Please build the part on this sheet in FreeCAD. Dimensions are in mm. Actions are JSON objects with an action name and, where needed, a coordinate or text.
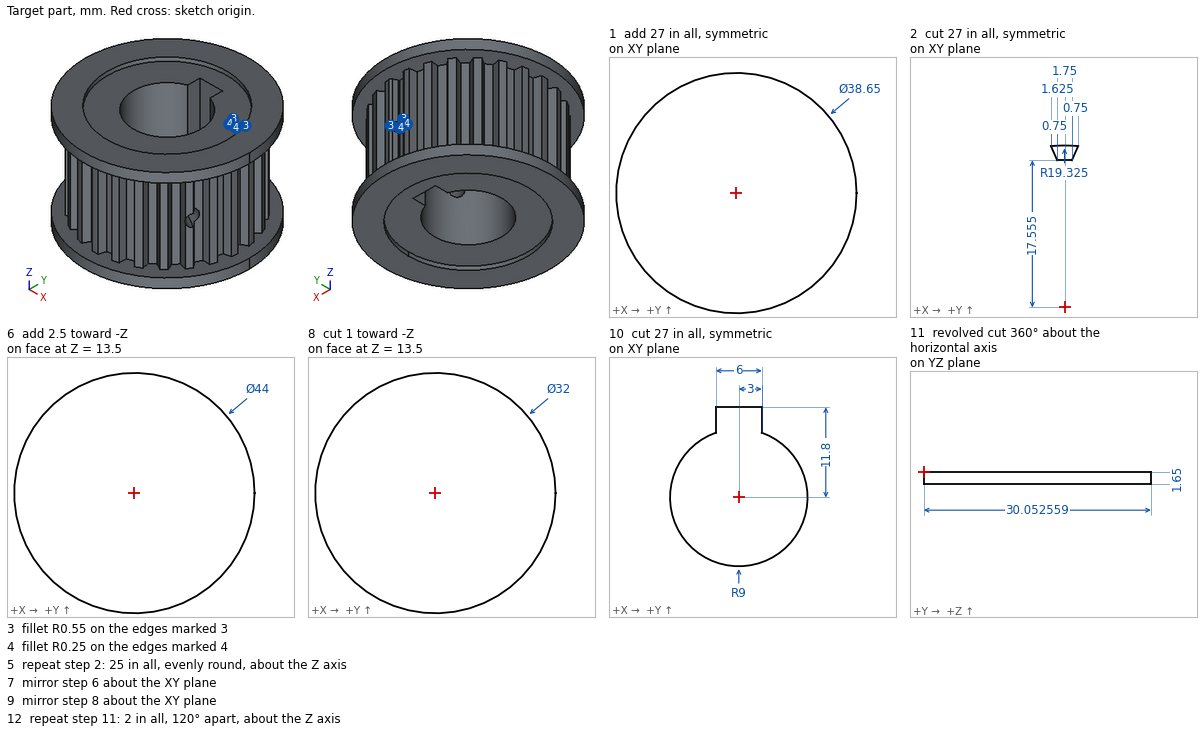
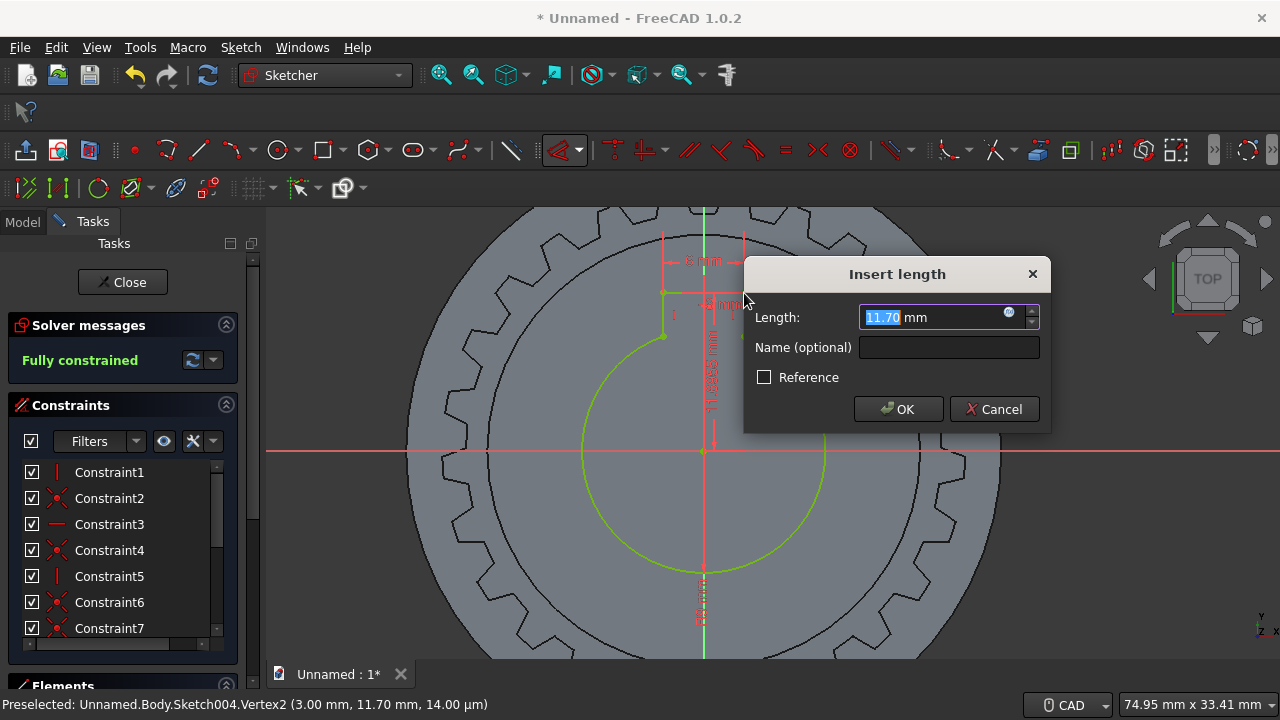
{"action": "type", "text": "11.8"}
{"action": "key", "text": "Return"}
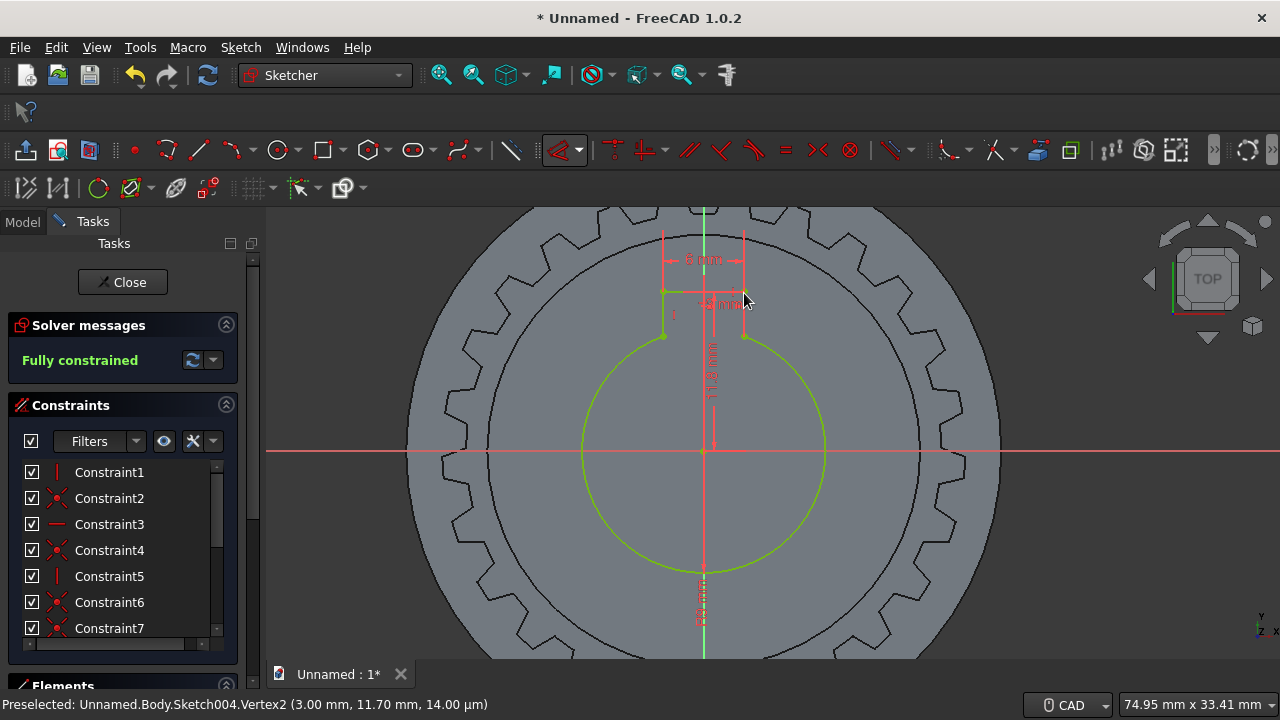
{"action": "left_click", "coordinate": [123, 282]}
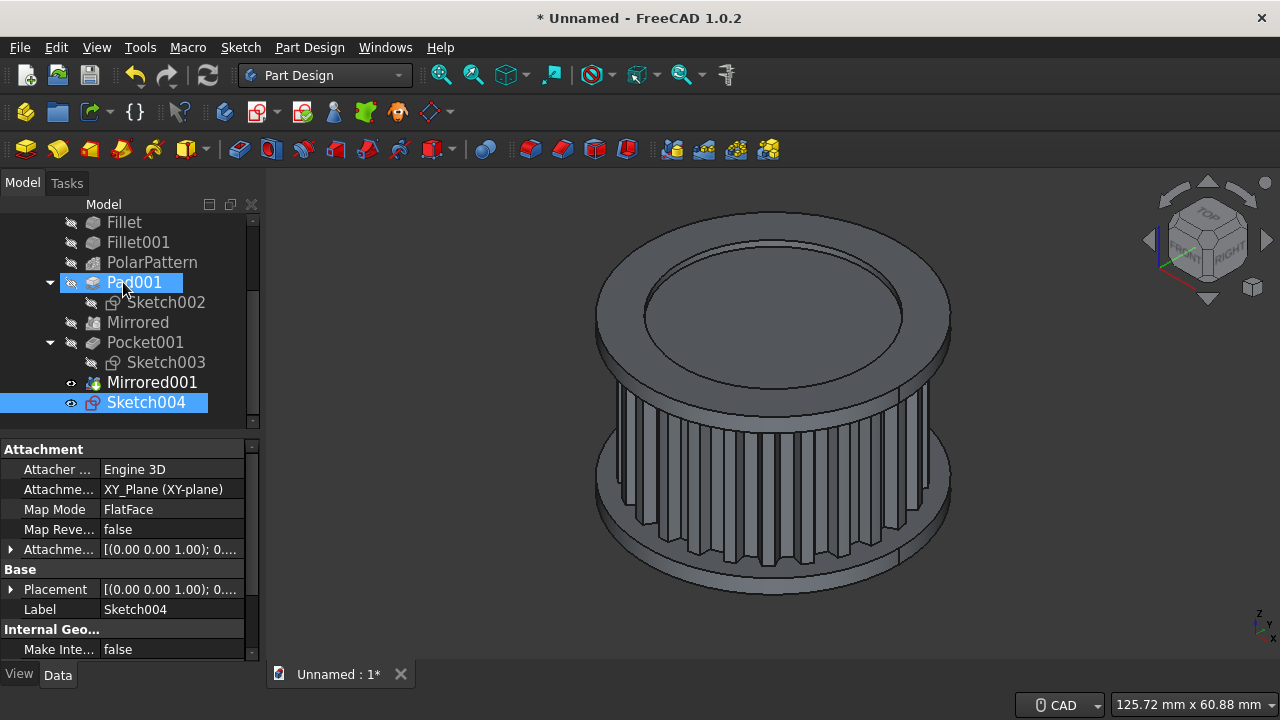
{"action": "left_click", "coordinate": [240, 150]}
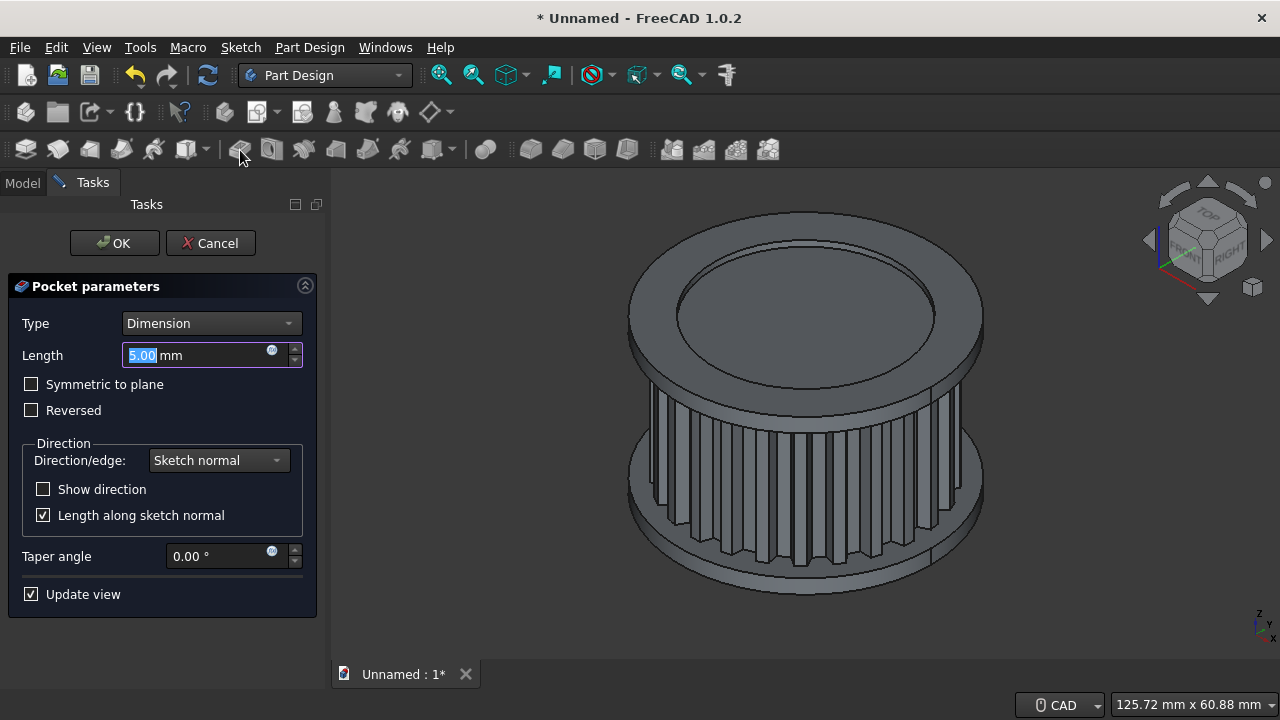
{"action": "type", "text": "27"}
{"action": "key", "text": "Tab"}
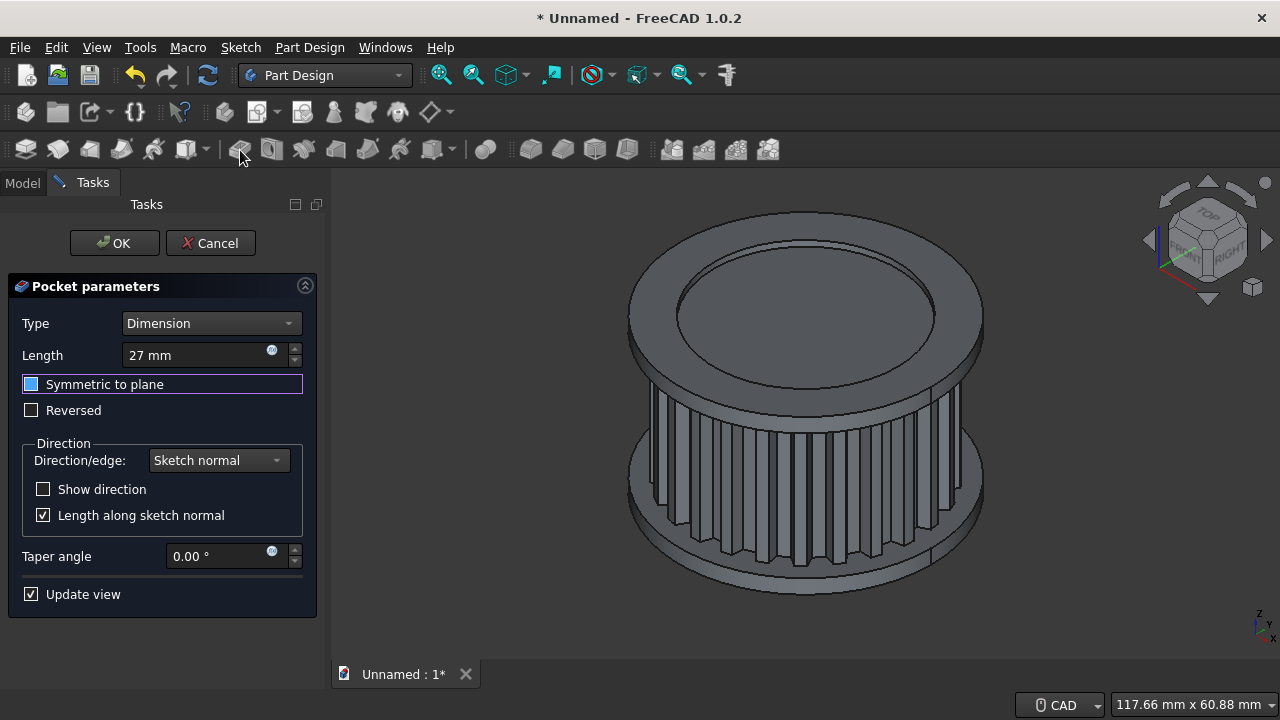
{"action": "left_click", "coordinate": [30, 384]}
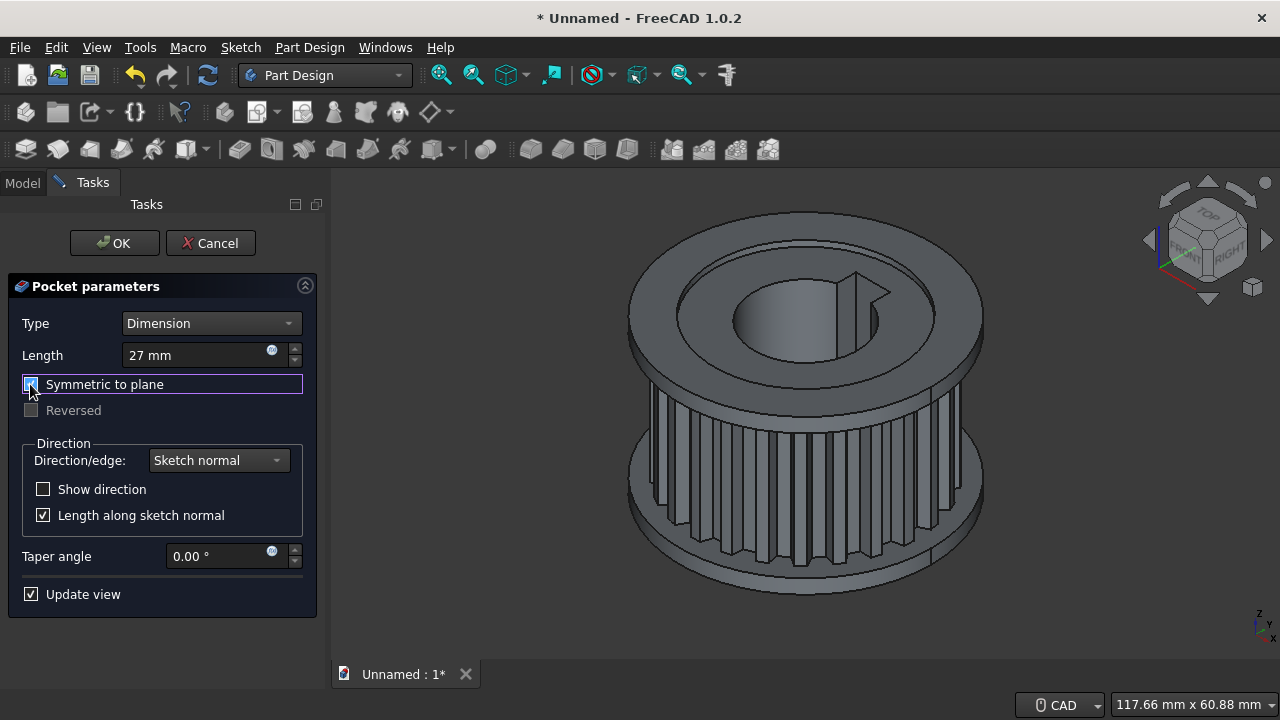
{"action": "left_click", "coordinate": [115, 243]}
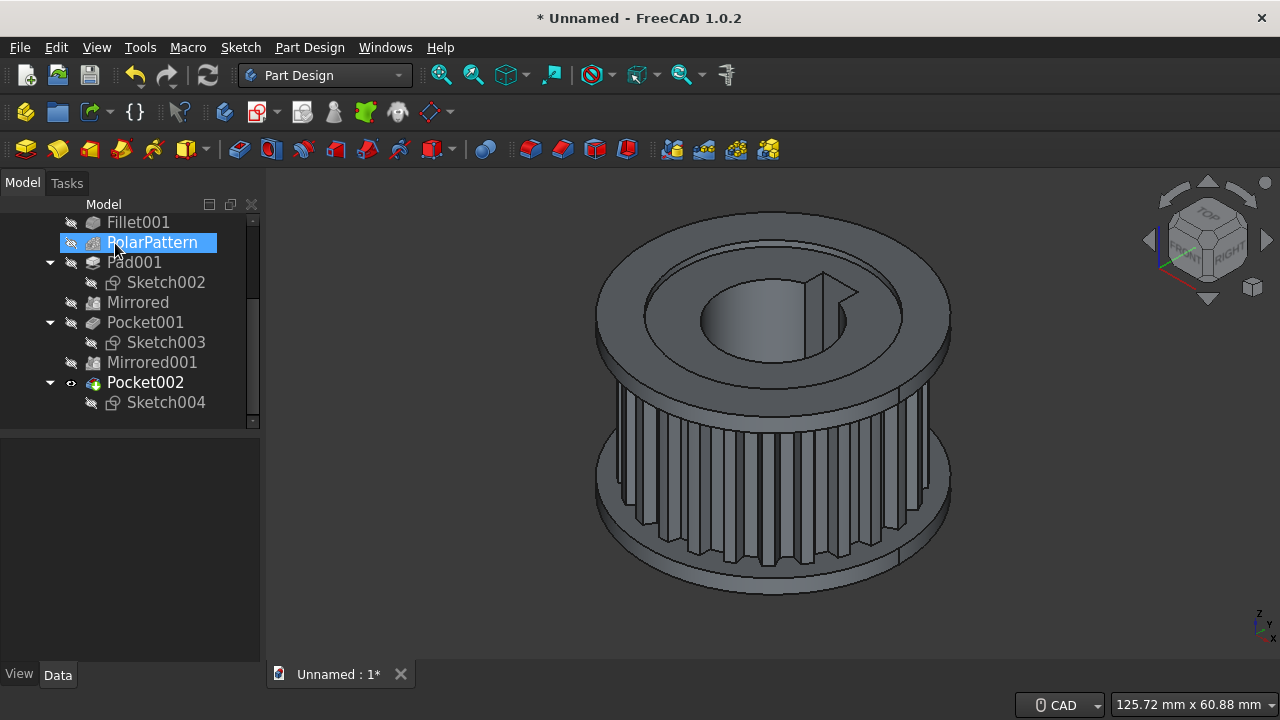
{"action": "left_click", "coordinate": [258, 112]}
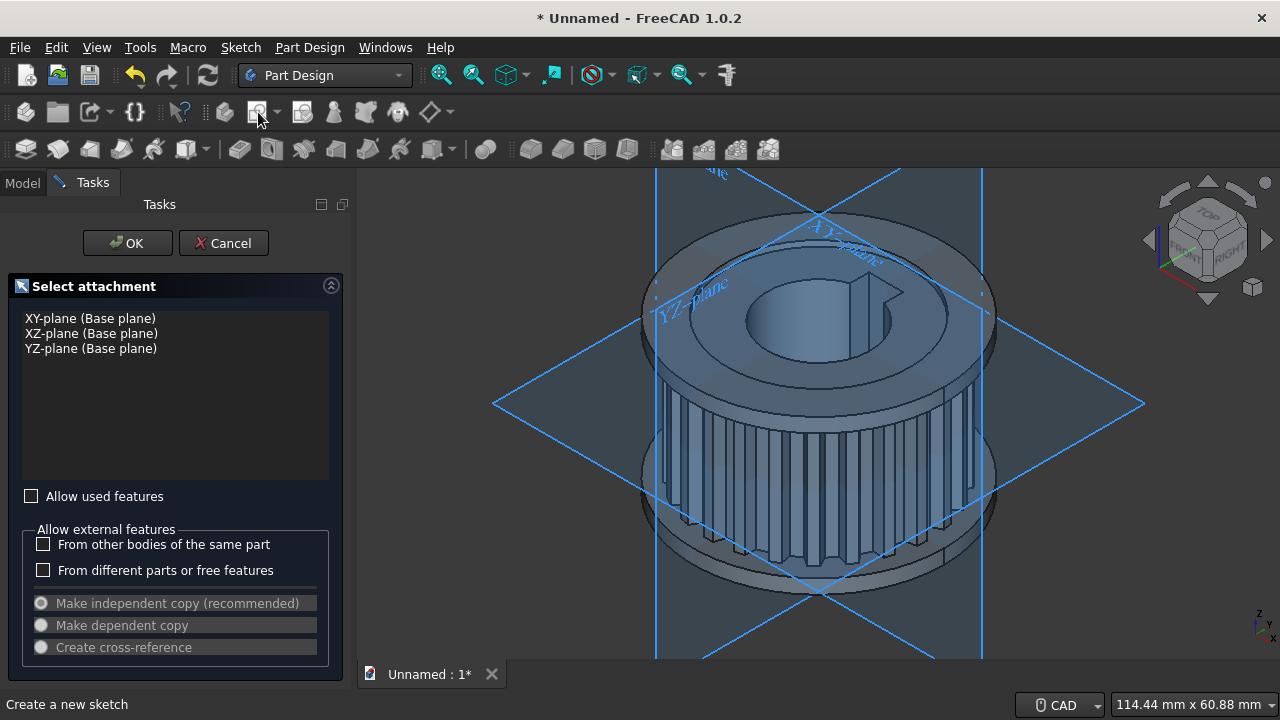
{"action": "left_click", "coordinate": [82, 348]}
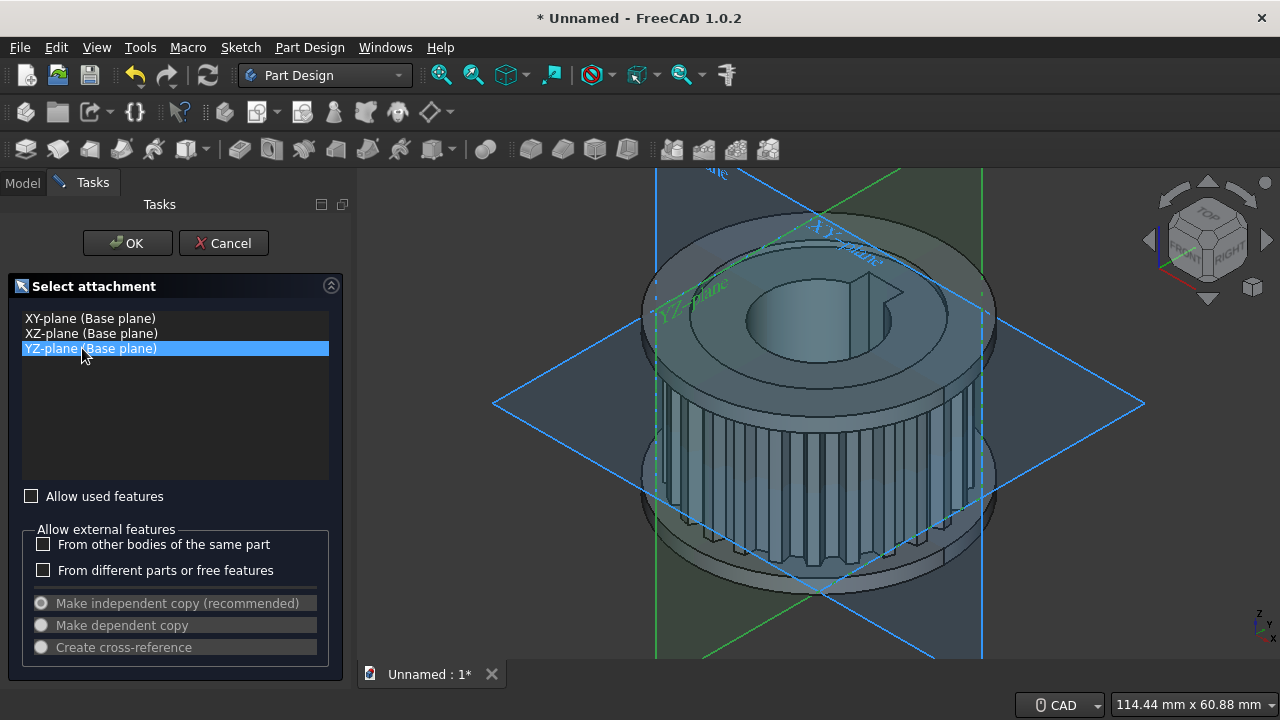
{"action": "left_click", "coordinate": [128, 243]}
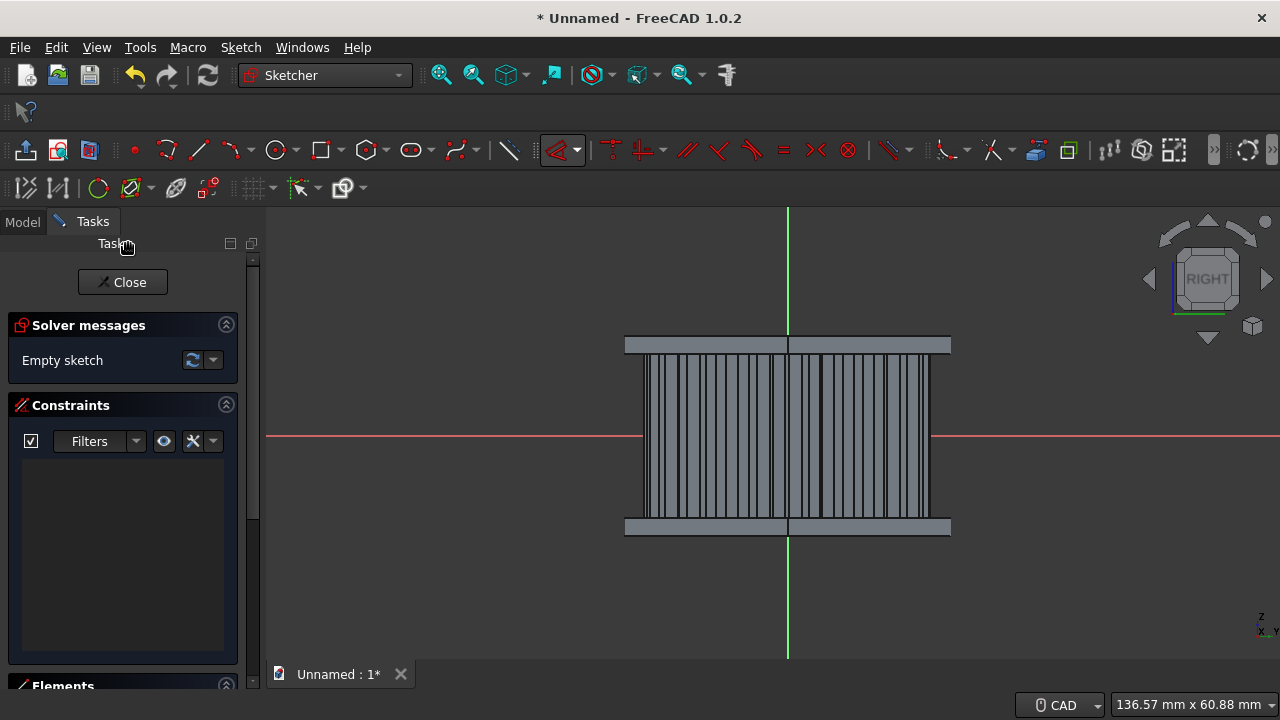
{"action": "left_click", "coordinate": [90, 150]}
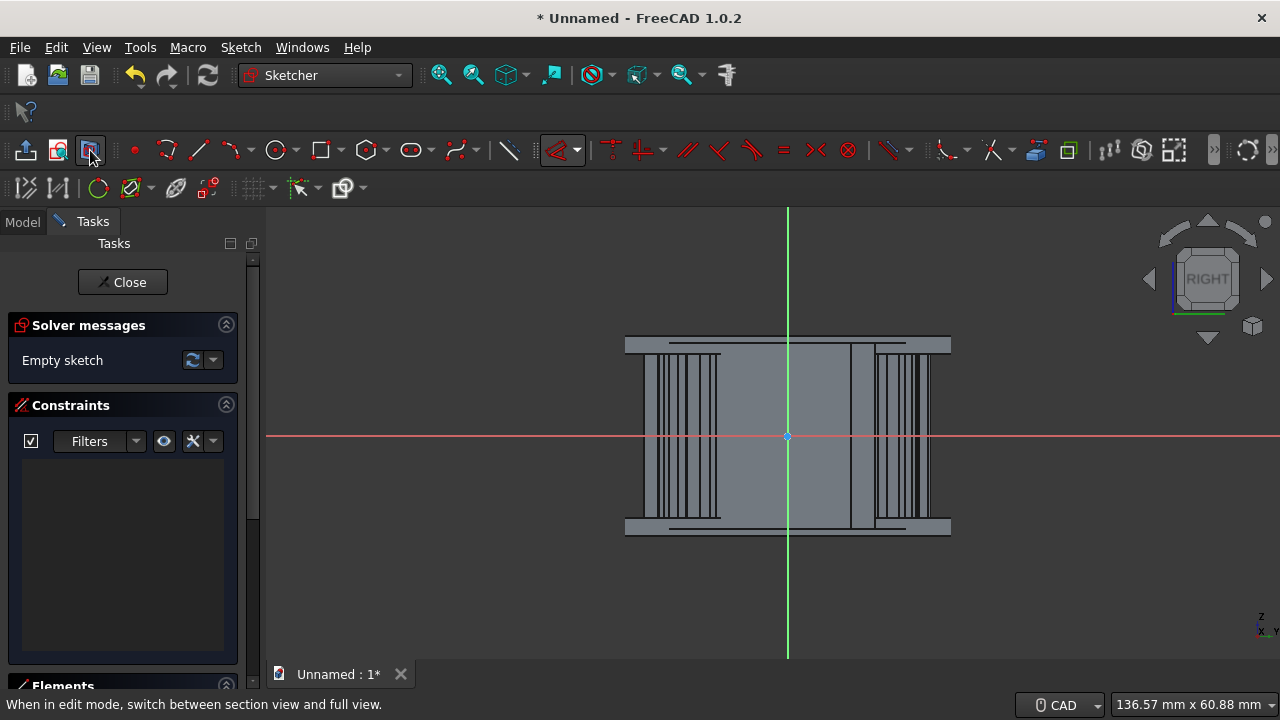
{"action": "scroll", "coordinate": [1013, 448], "scroll_direction": "up", "scroll_amount": 5}